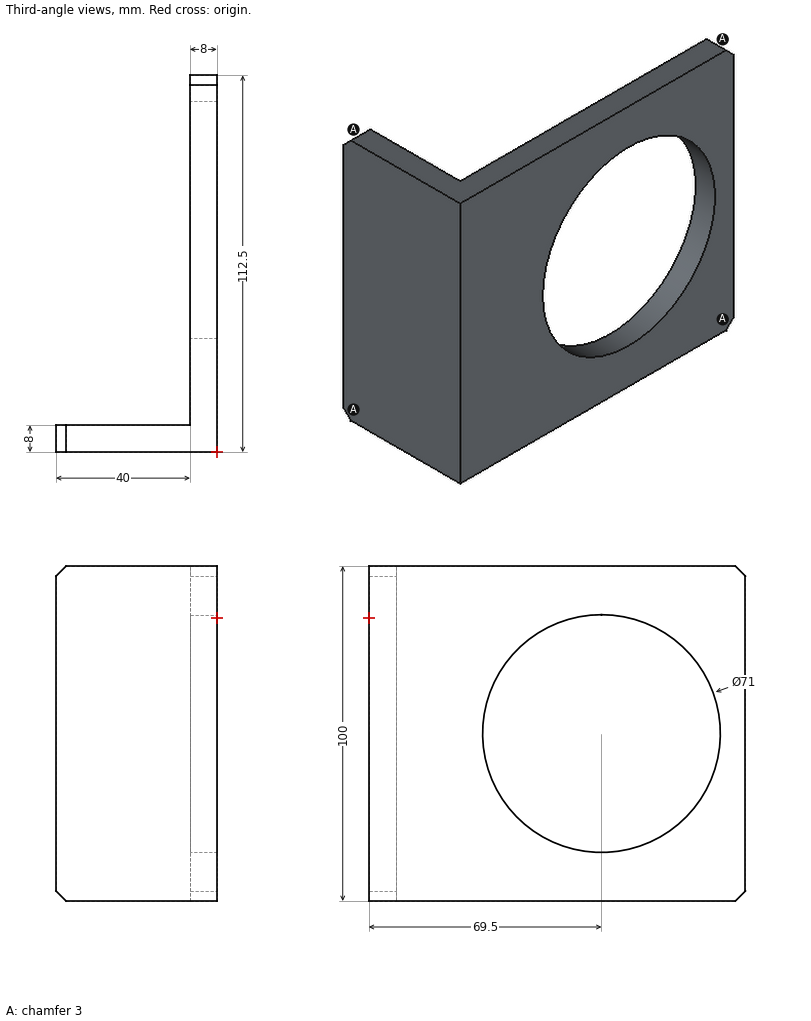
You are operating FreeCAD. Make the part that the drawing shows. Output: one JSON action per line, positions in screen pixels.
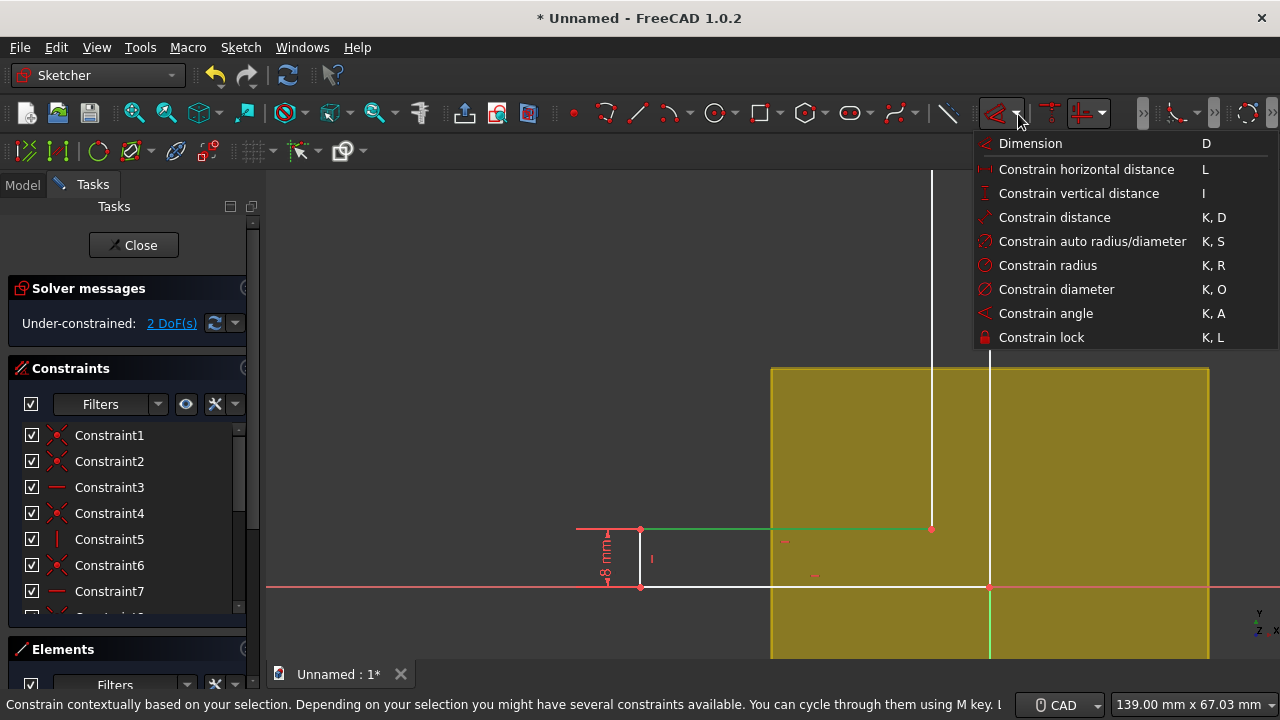
{"action": "left_click", "coordinate": [1126, 169]}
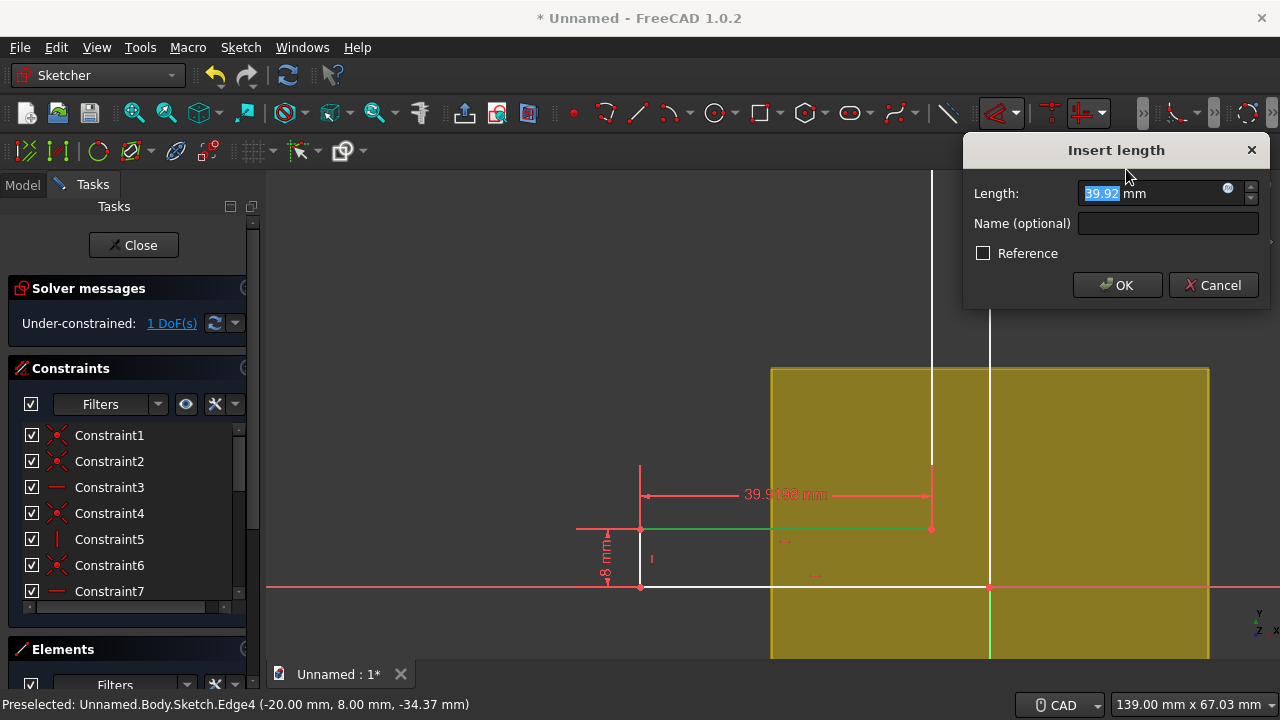
{"action": "type", "text": "40"}
{"action": "key", "text": "Return"}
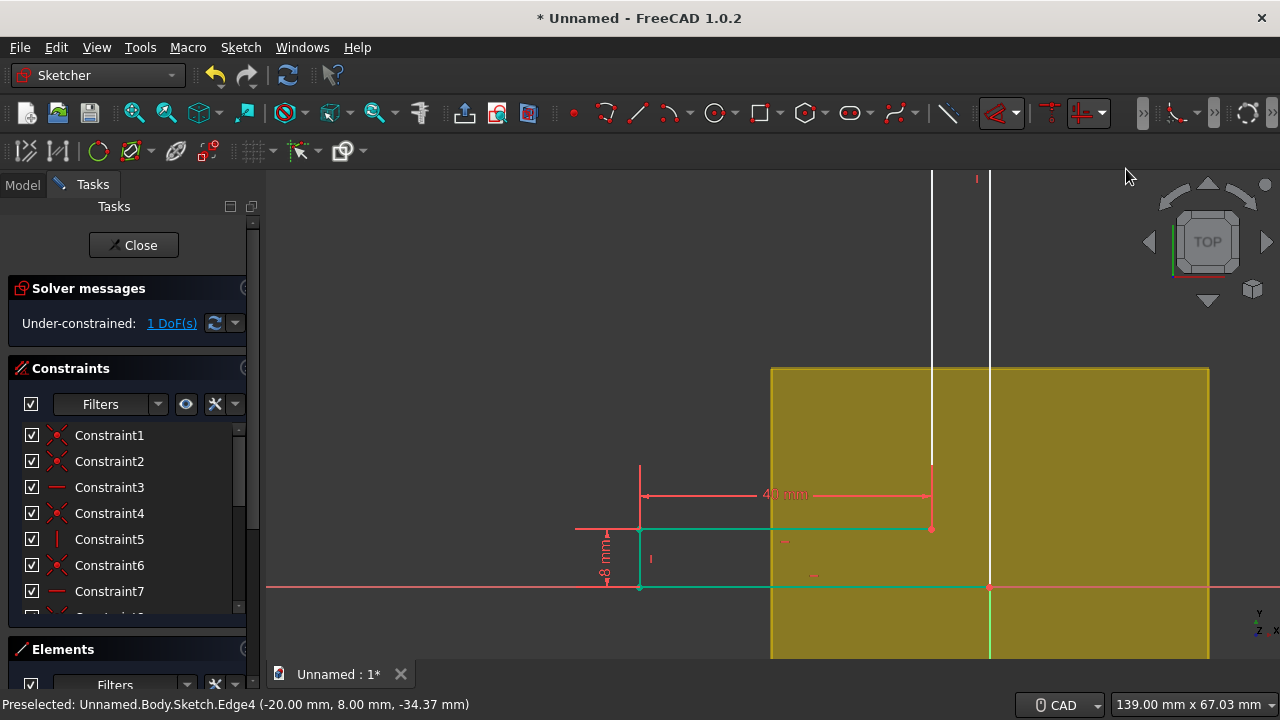
{"action": "left_click", "coordinate": [990, 342]}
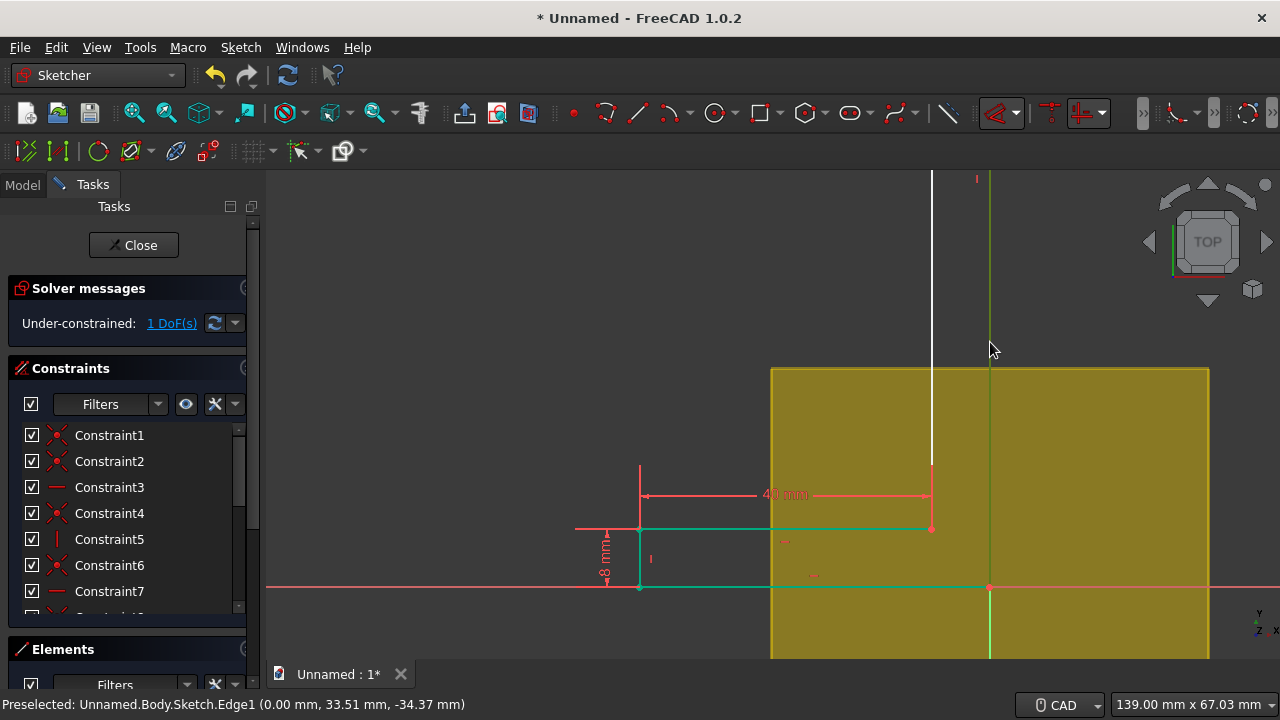
{"action": "left_click", "coordinate": [1018, 114]}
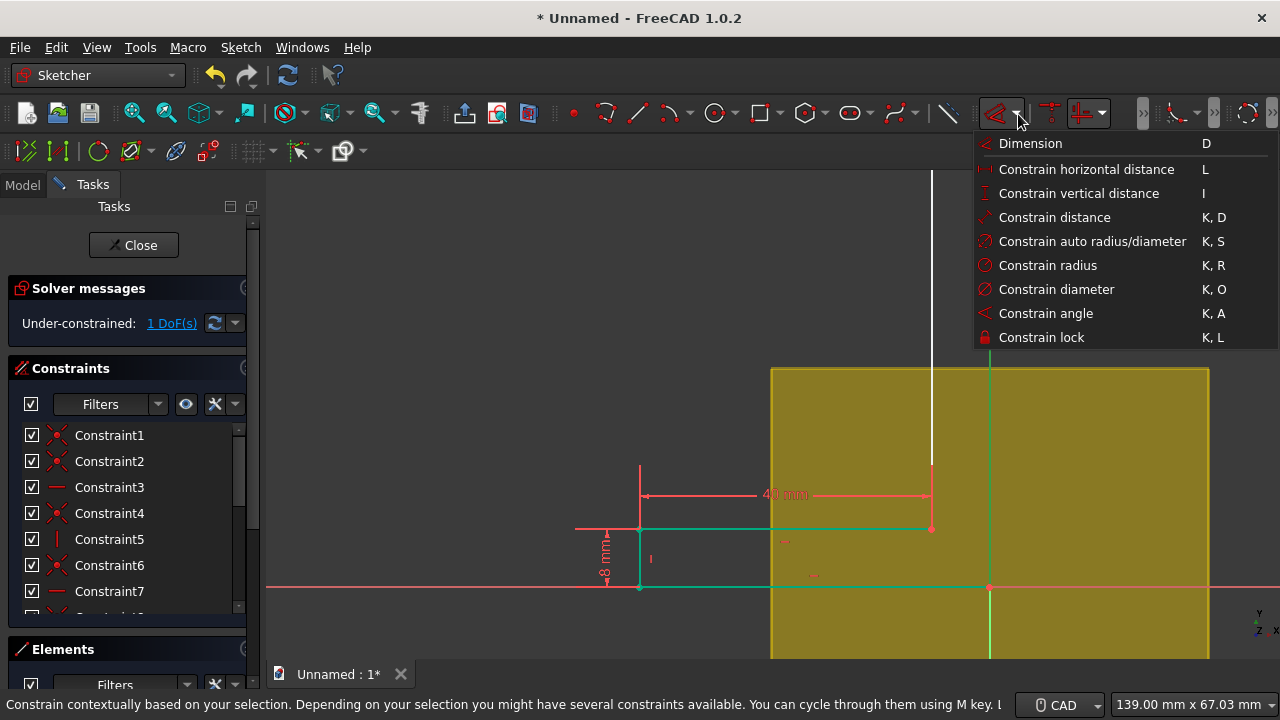
{"action": "left_click", "coordinate": [1126, 193]}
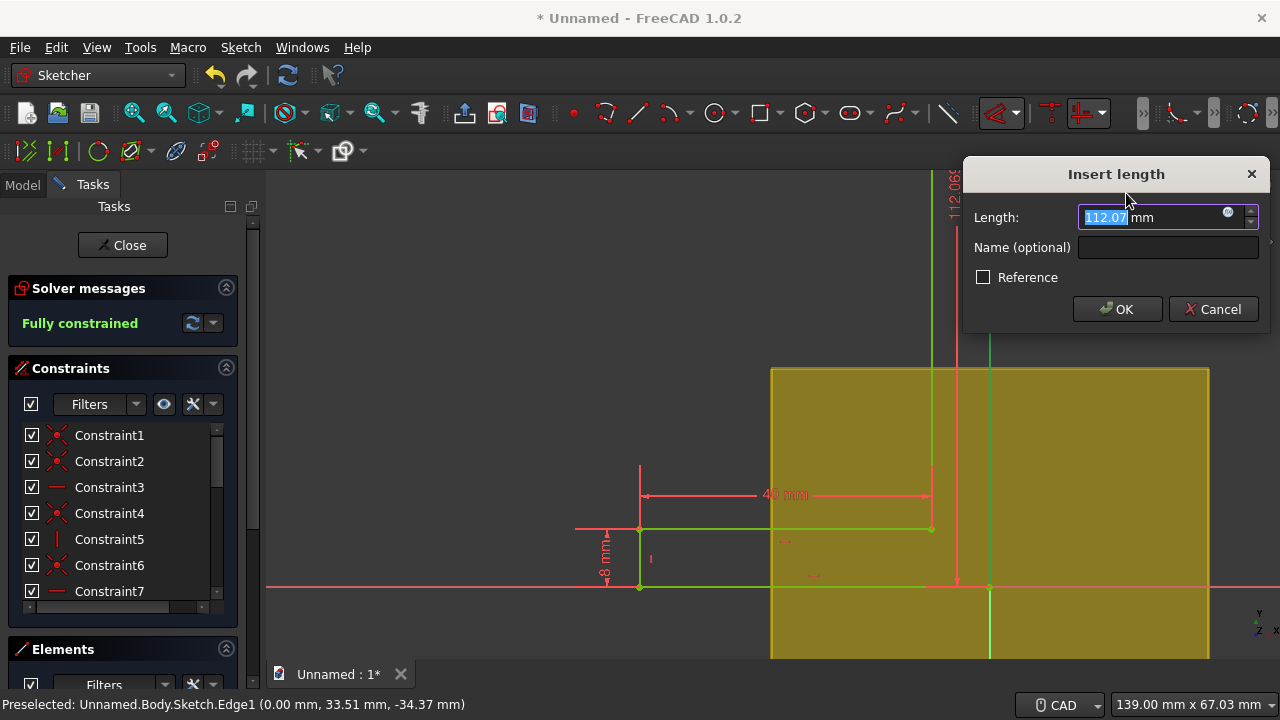
{"action": "type", "text": "112.5"}
{"action": "key", "text": "Return"}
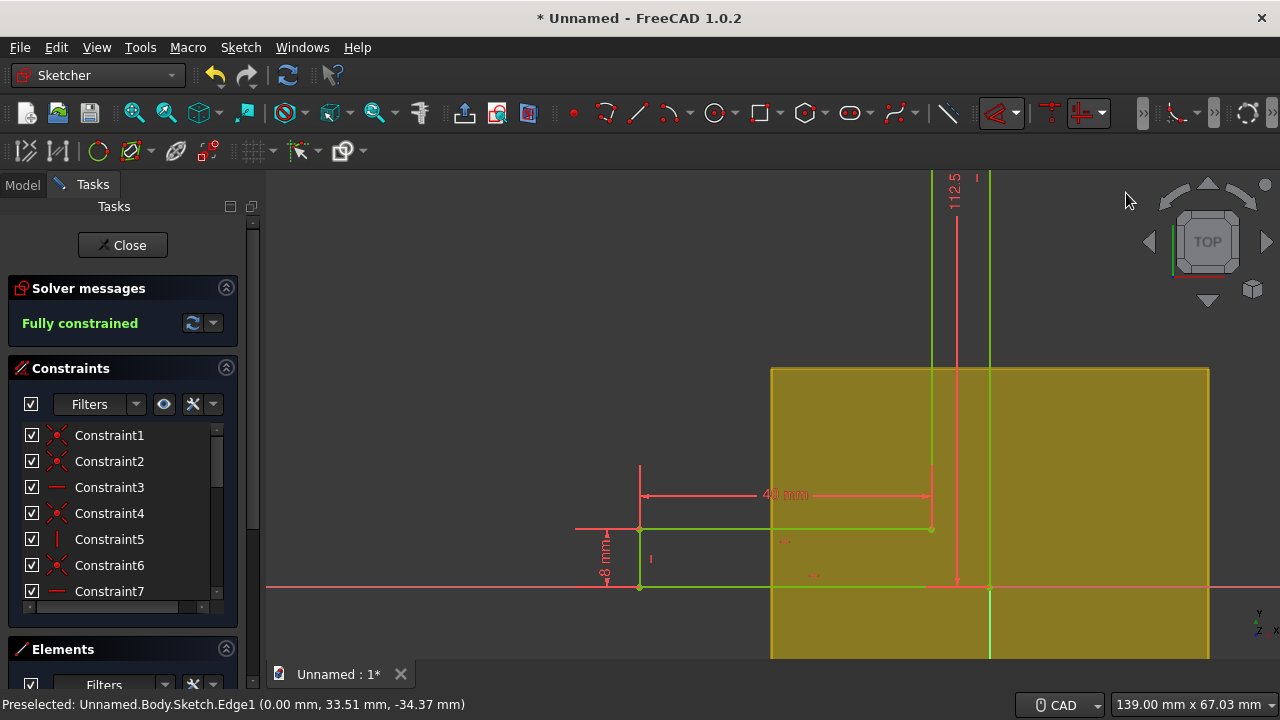
{"action": "left_click", "coordinate": [123, 245]}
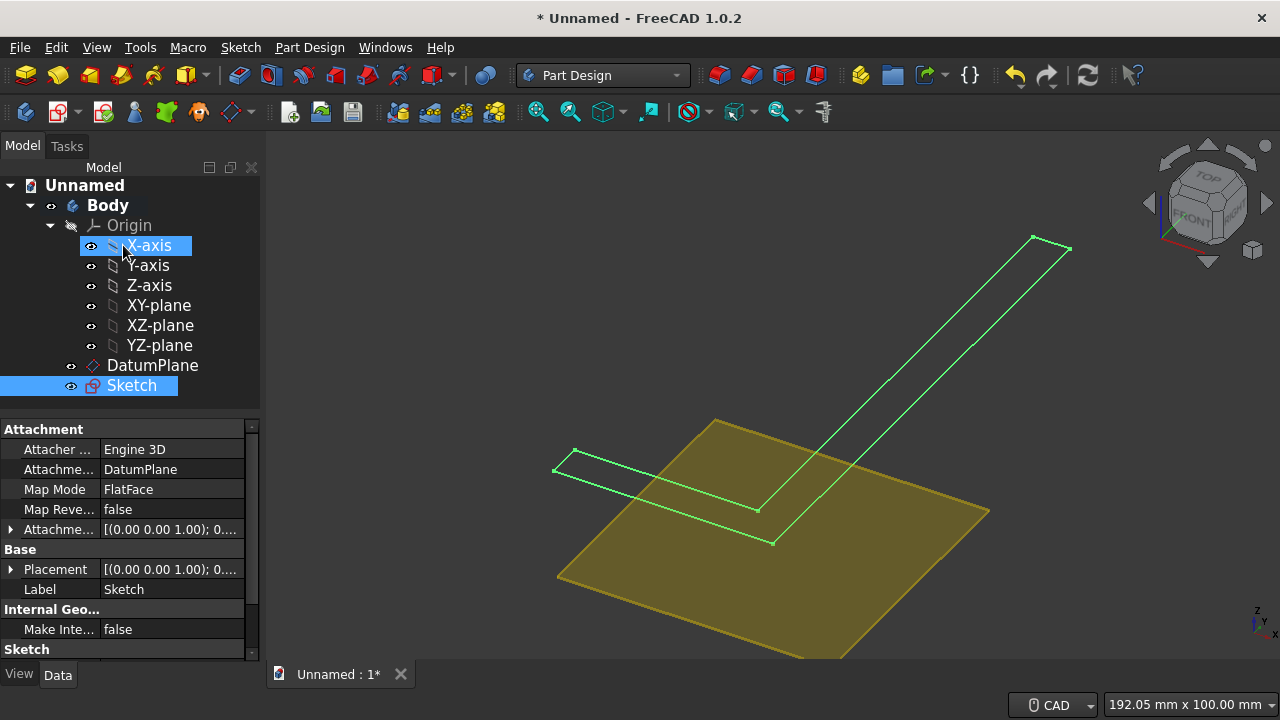
{"action": "left_click", "coordinate": [26, 76]}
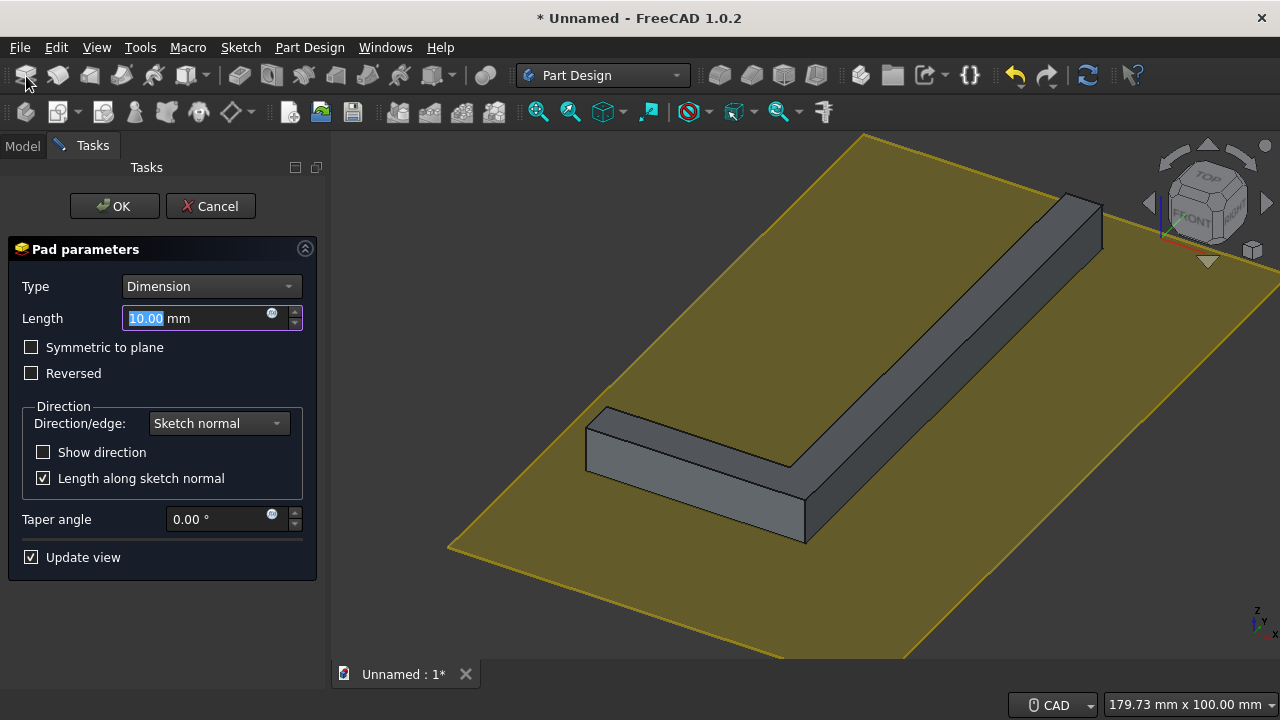
{"action": "type", "text": "100"}
{"action": "key", "text": "Tab"}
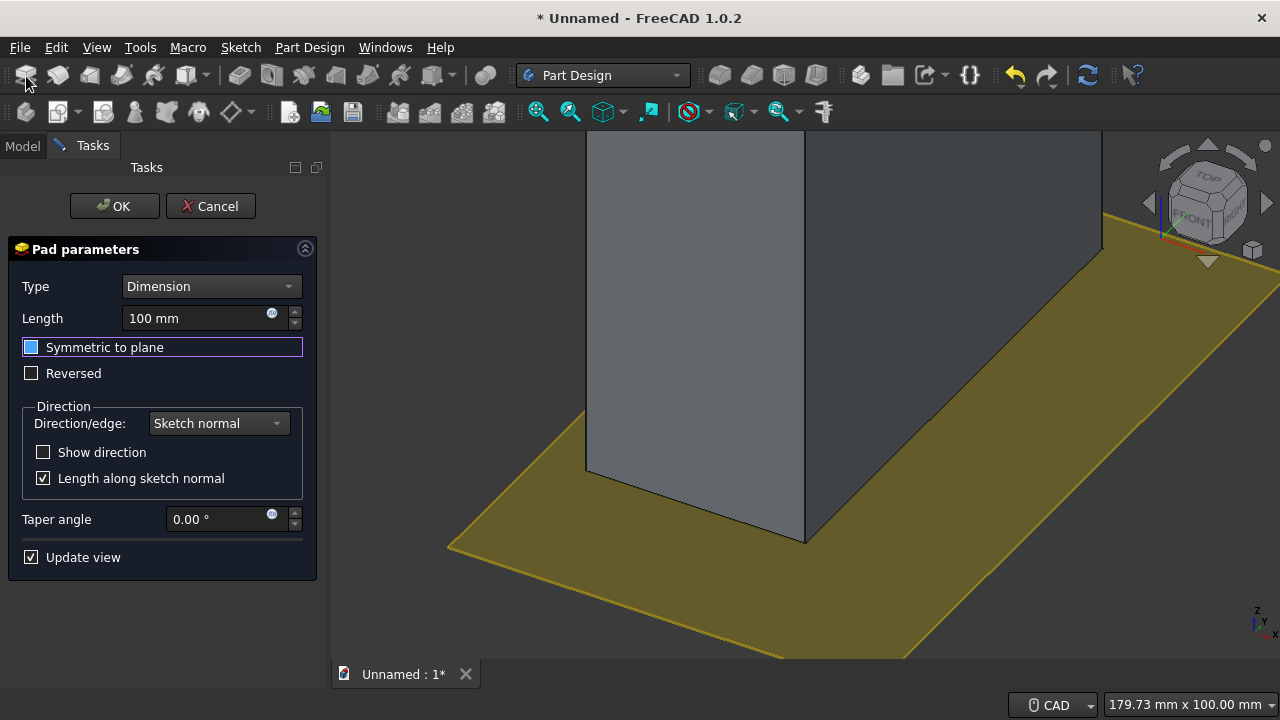
{"action": "left_click", "coordinate": [30, 347]}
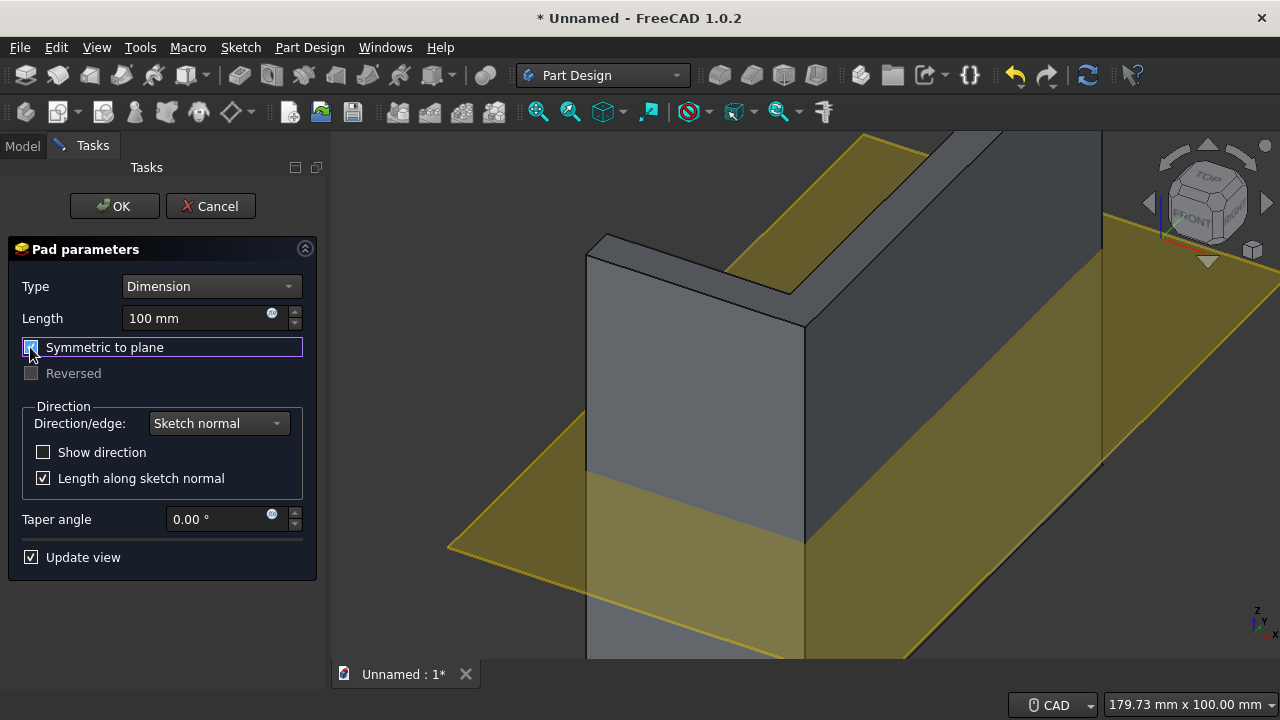
{"action": "left_click", "coordinate": [115, 206]}